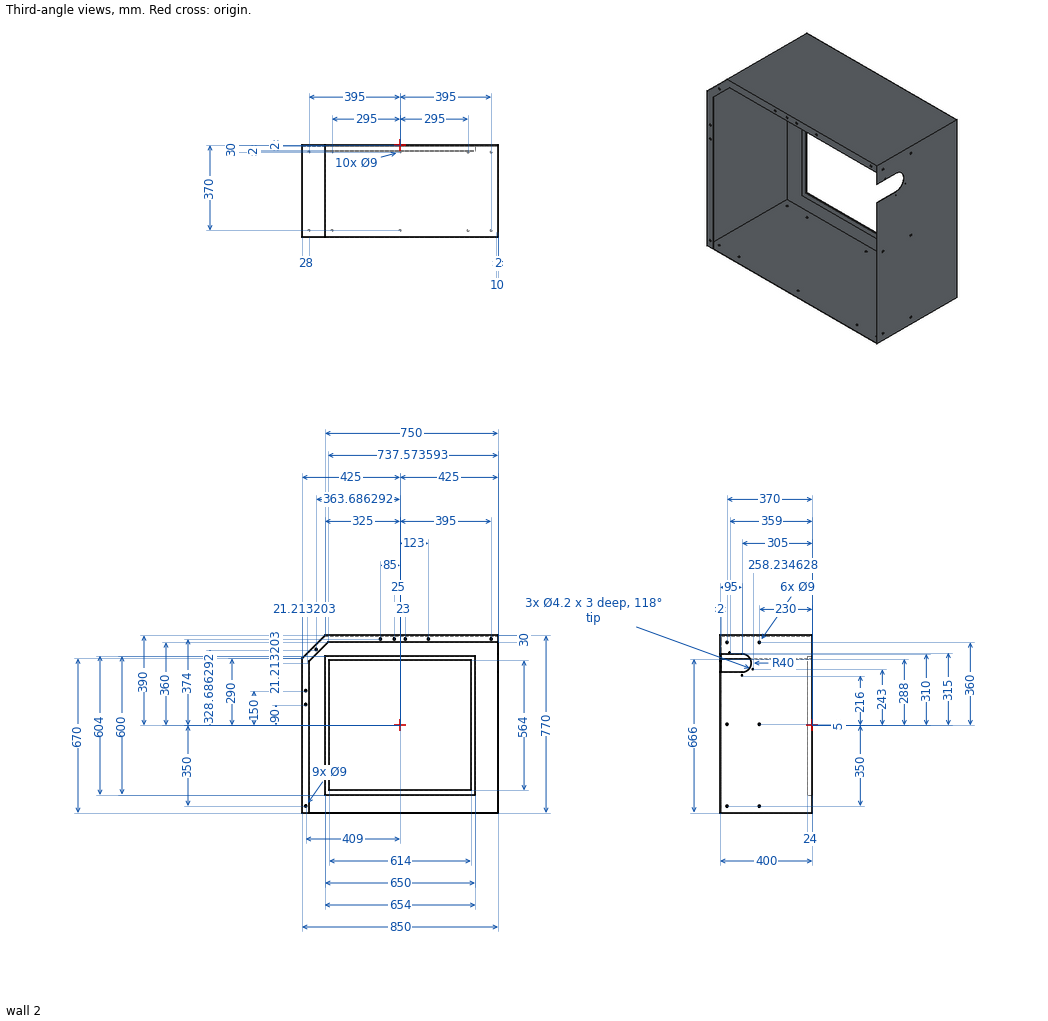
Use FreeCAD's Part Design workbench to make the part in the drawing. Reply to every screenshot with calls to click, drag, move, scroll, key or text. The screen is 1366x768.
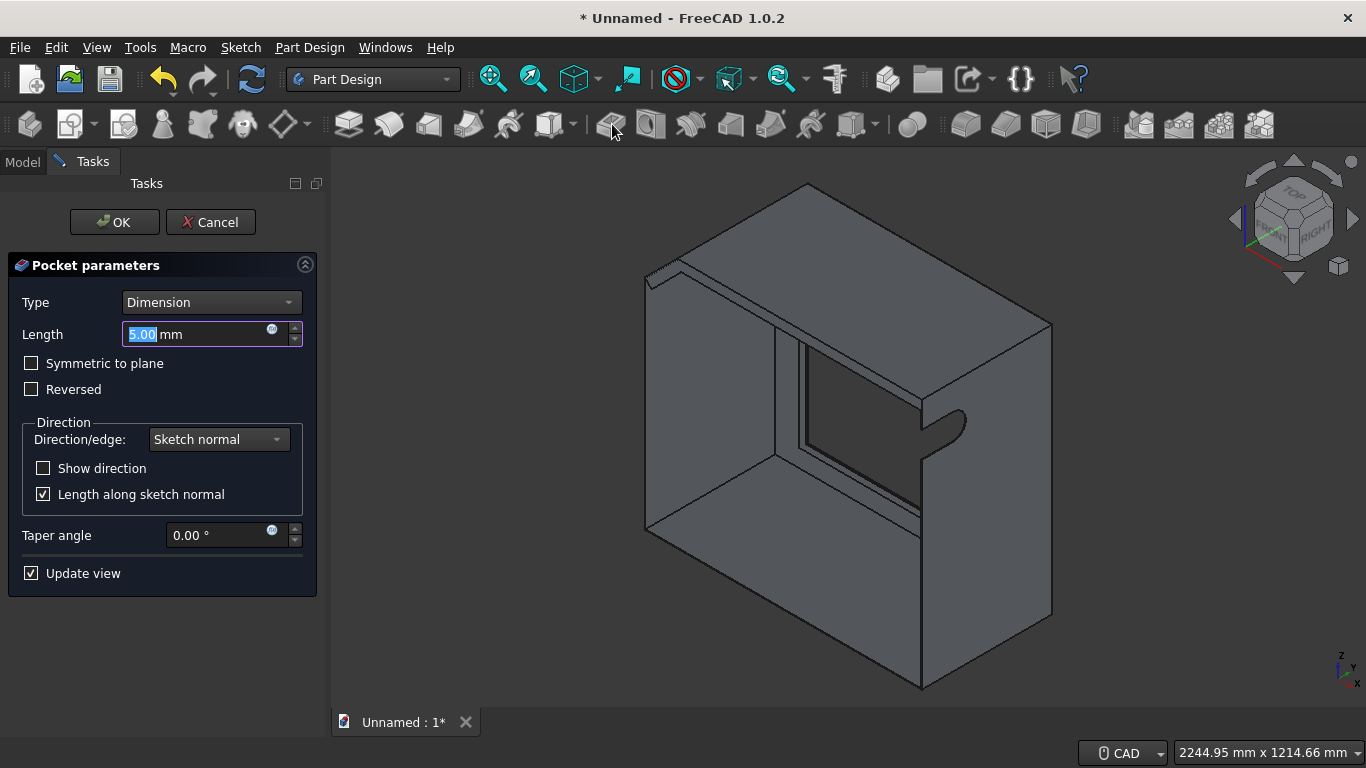
text(2)
key(Tab)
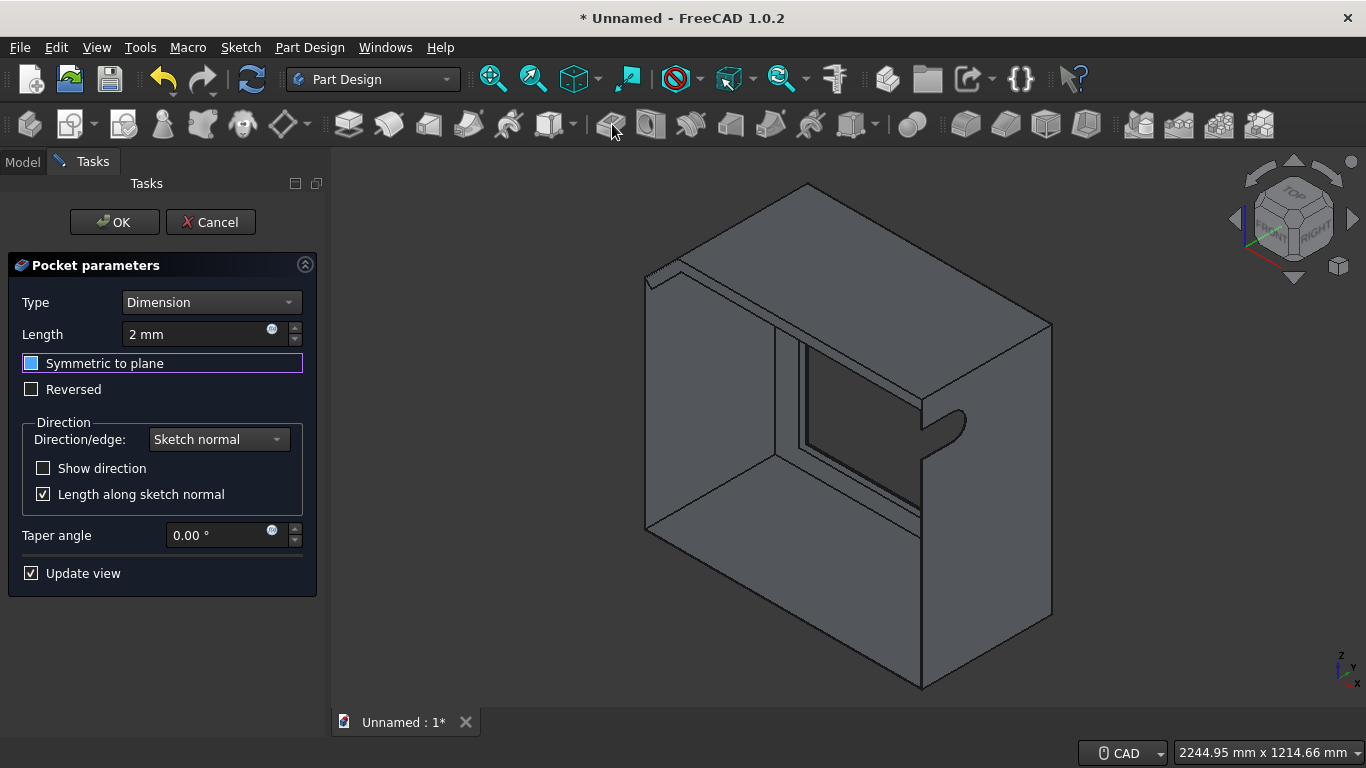
click(115, 222)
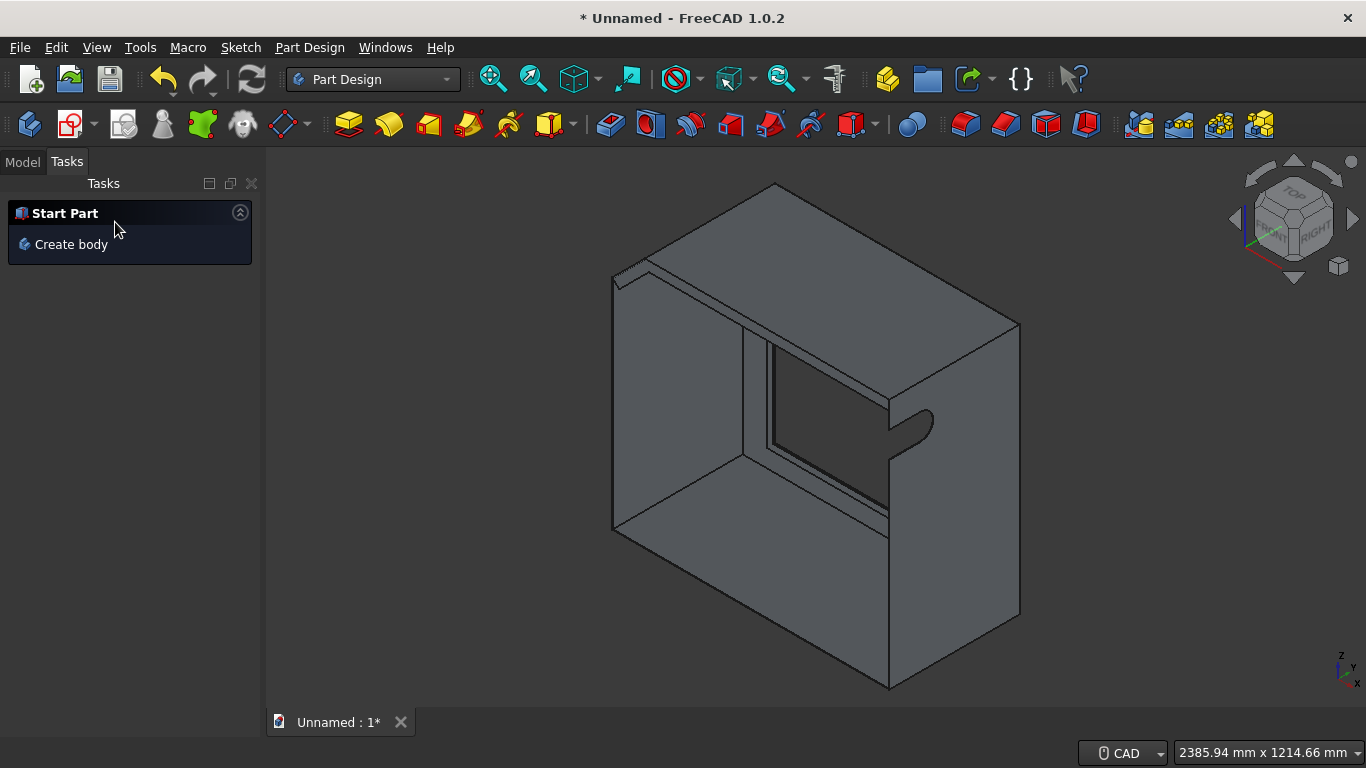
click(23, 161)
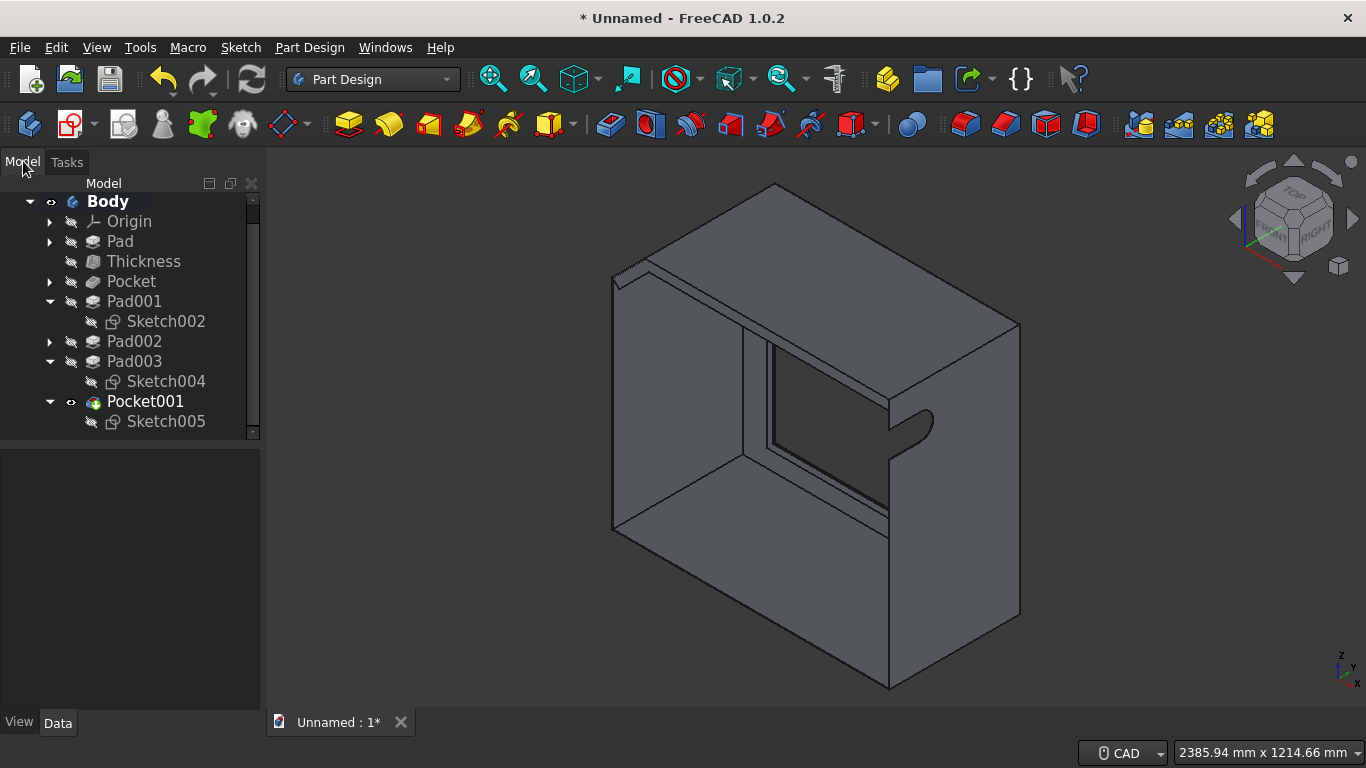
click(50, 222)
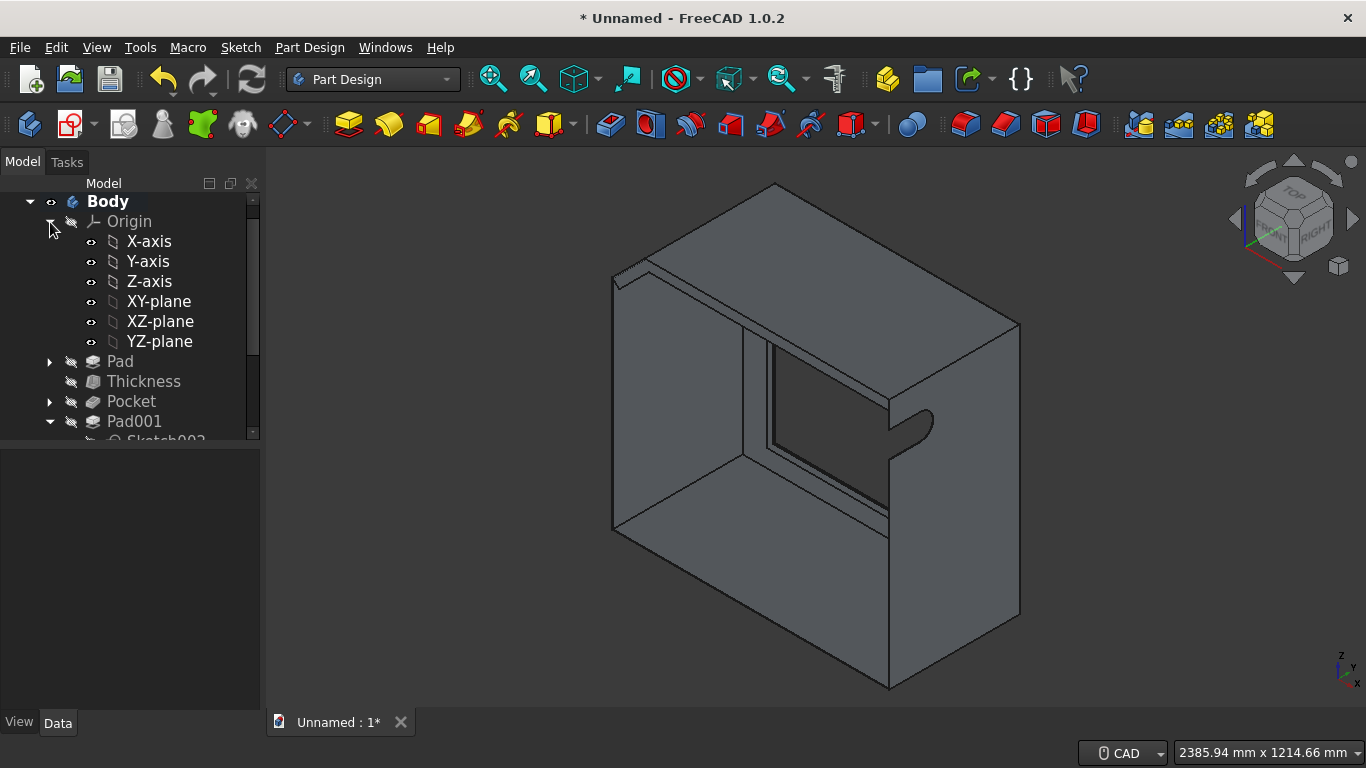
click(136, 342)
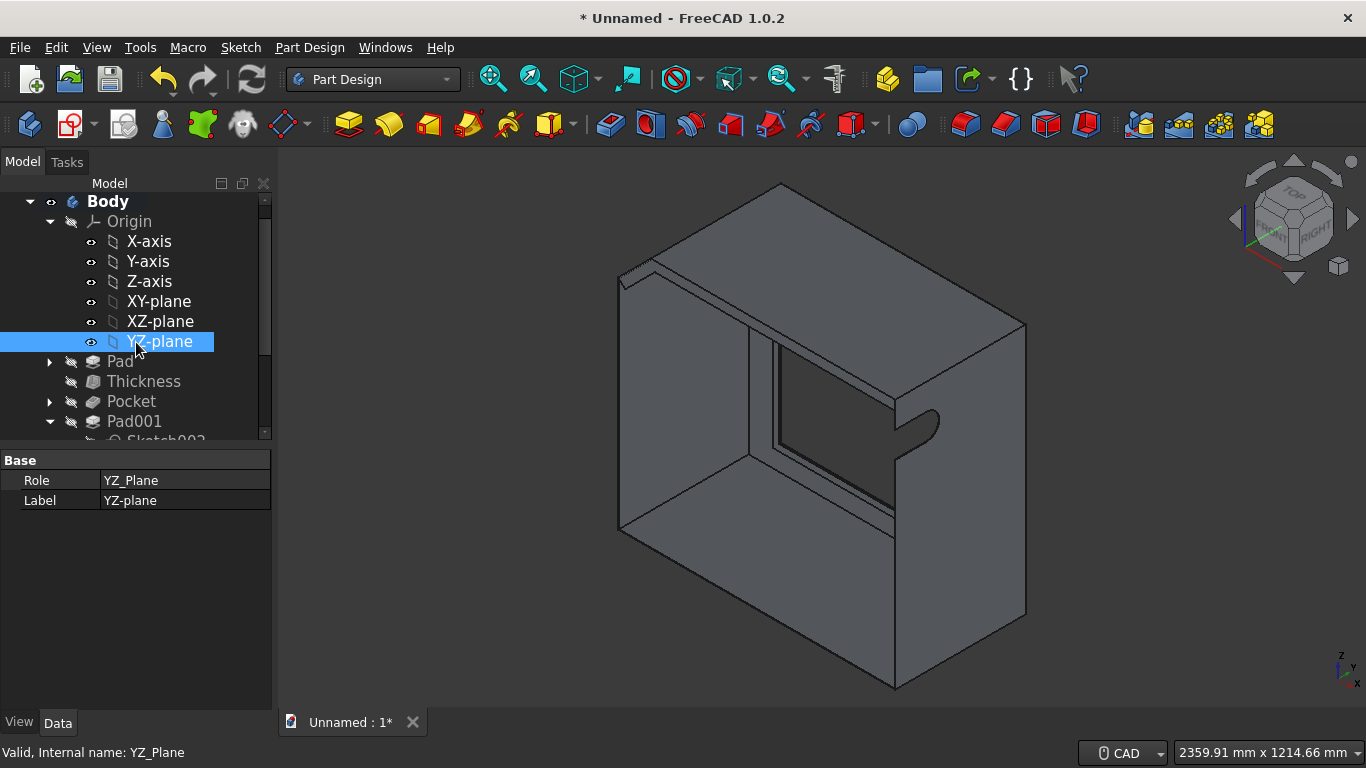
click(284, 124)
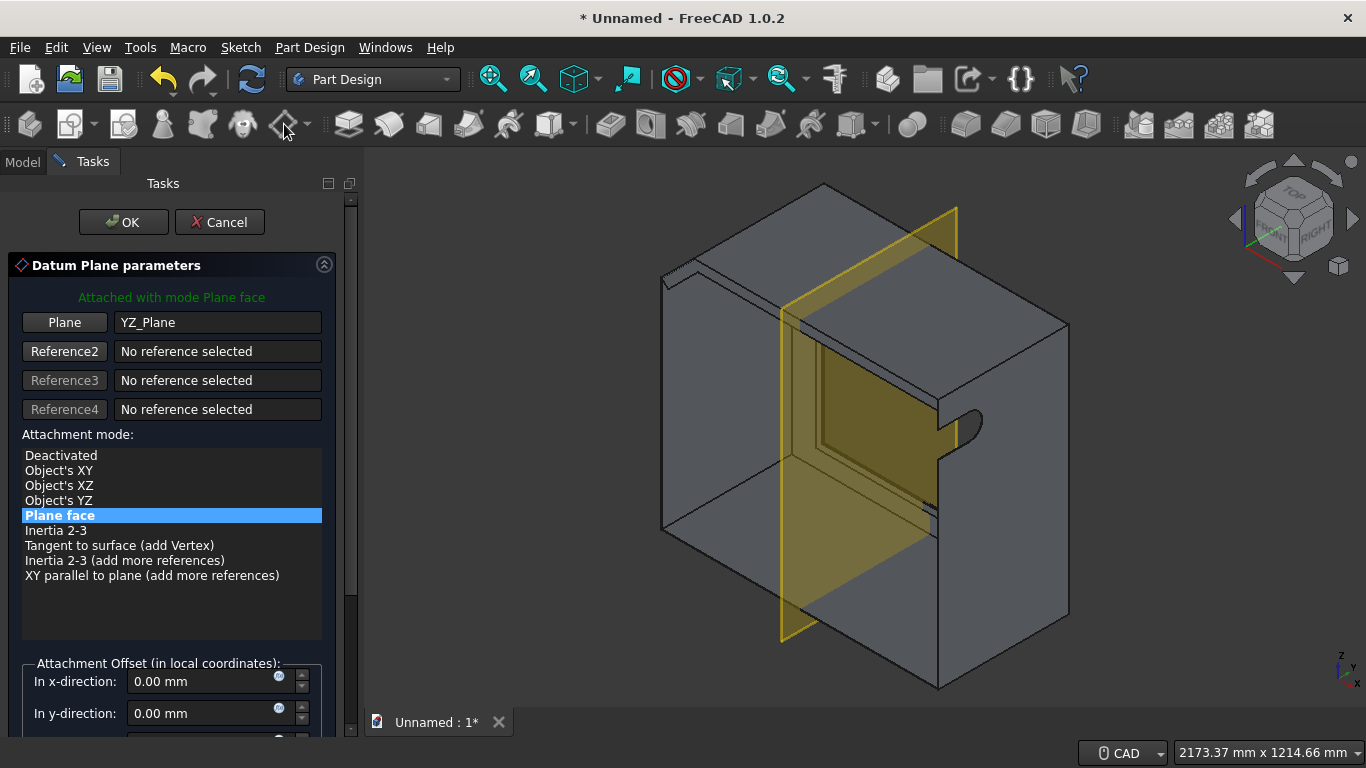
scroll(351, 464, down, 2)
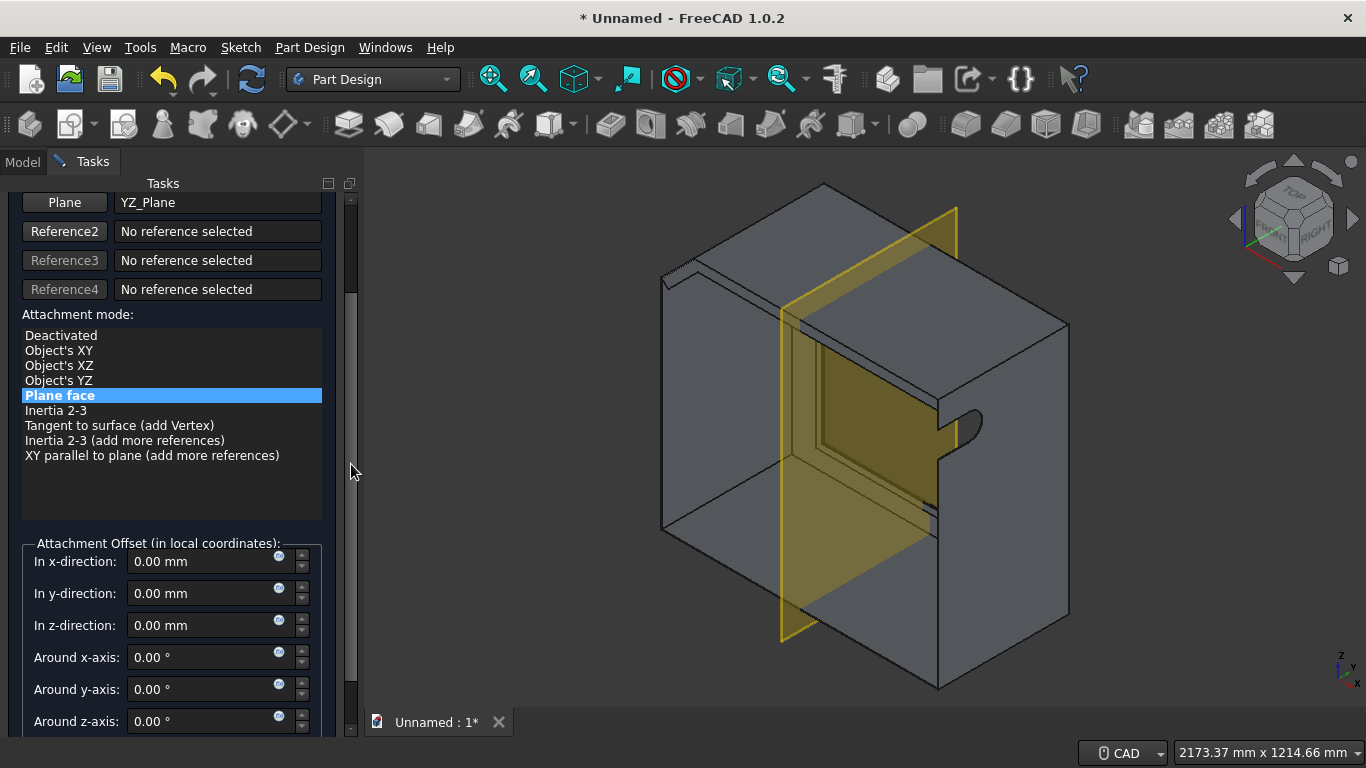
triple_click(210, 625)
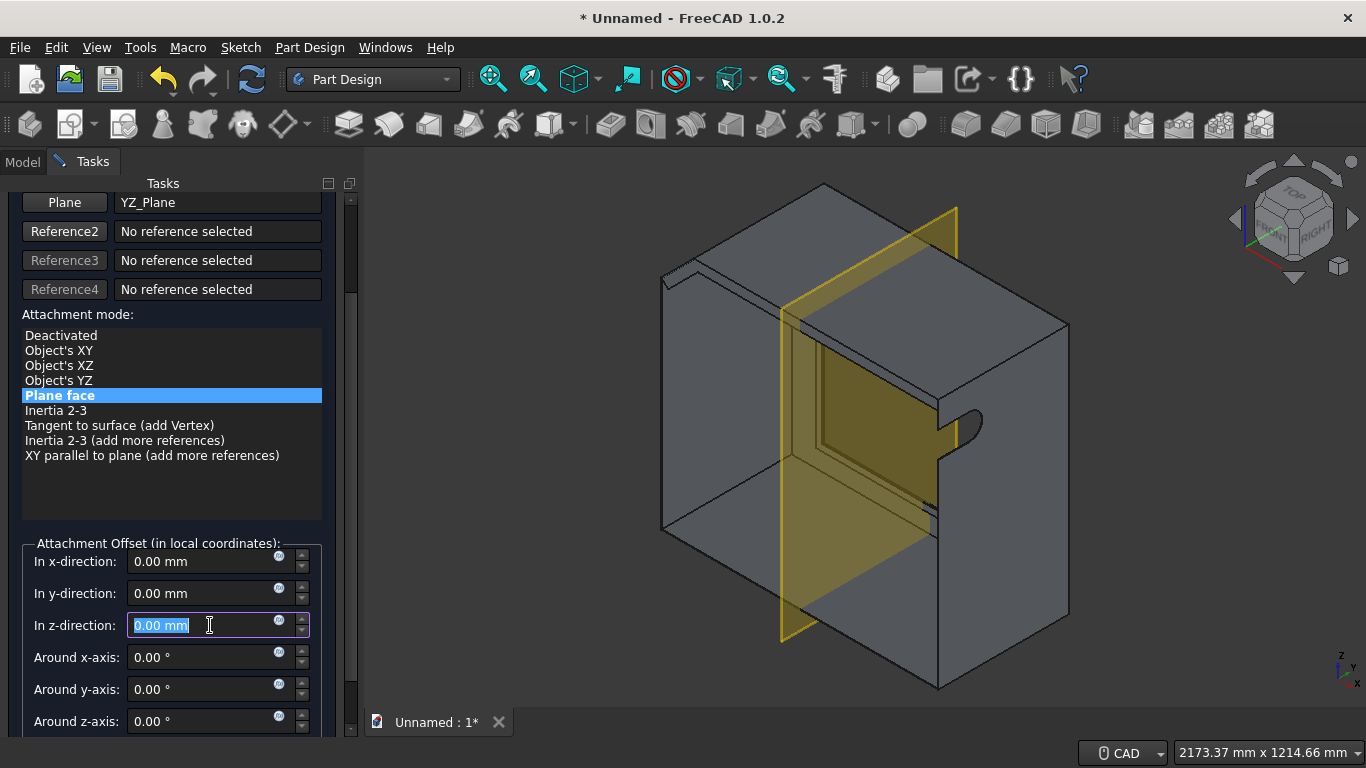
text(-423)
key(Tab)